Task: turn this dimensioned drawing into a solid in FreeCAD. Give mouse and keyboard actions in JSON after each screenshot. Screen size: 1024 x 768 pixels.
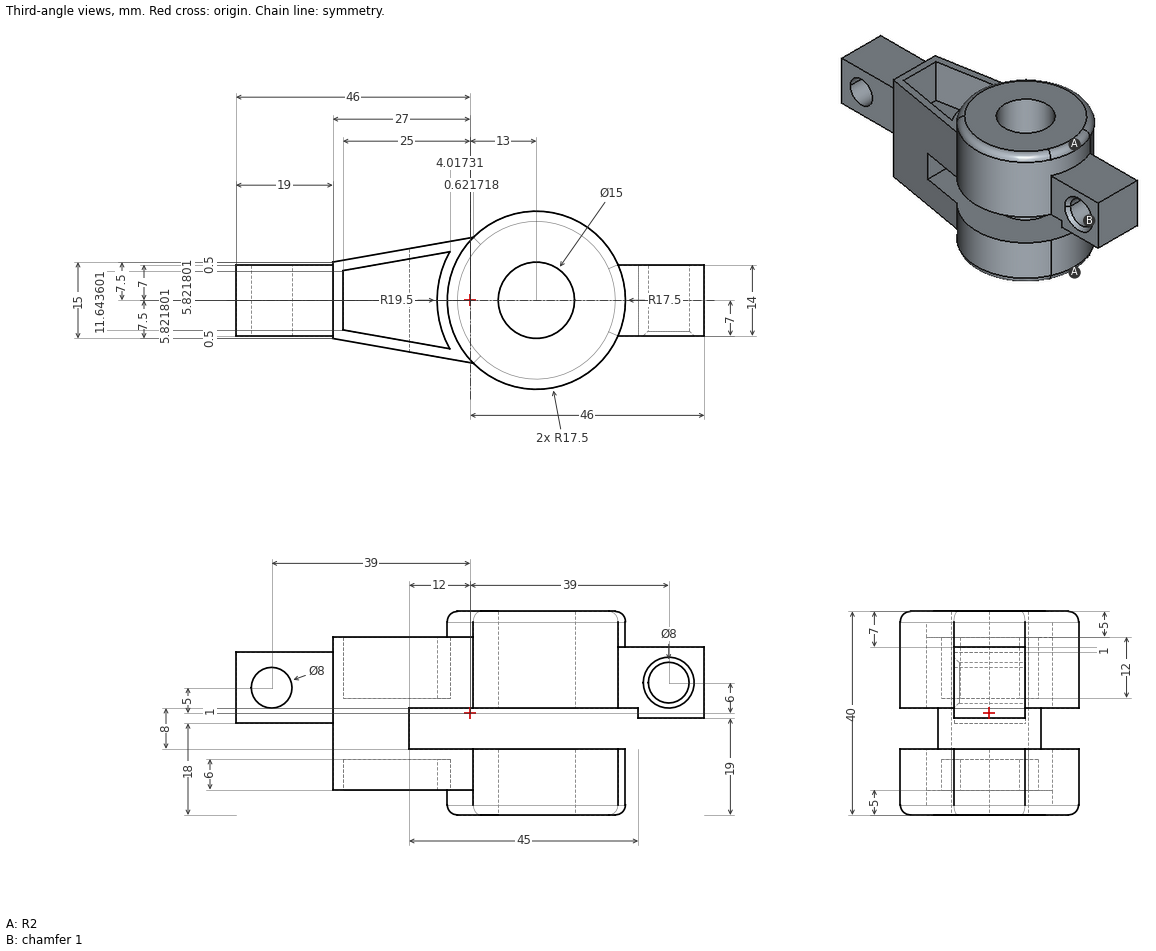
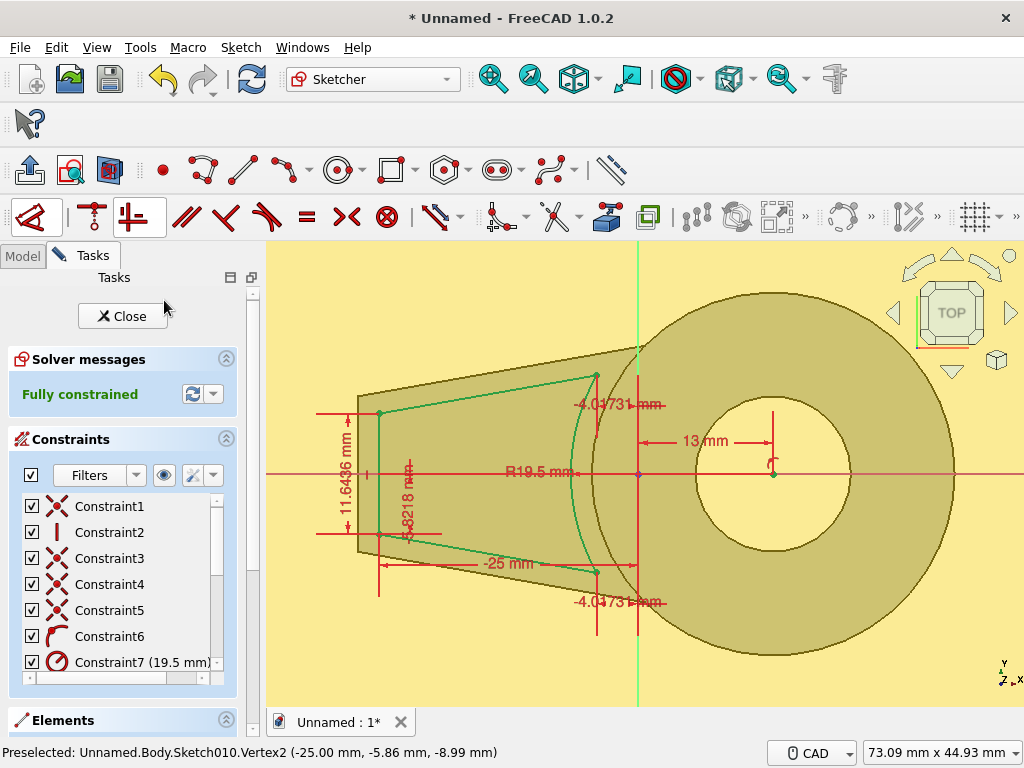
{"action": "left_click", "coordinate": [123, 316]}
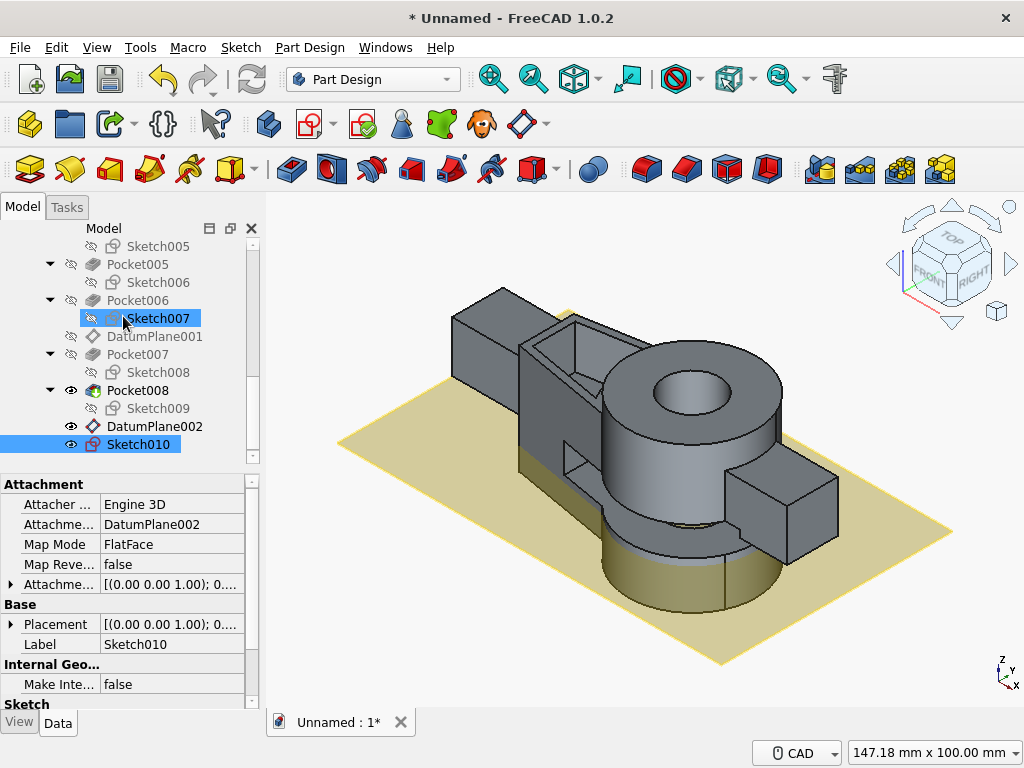
{"action": "left_click", "coordinate": [292, 170]}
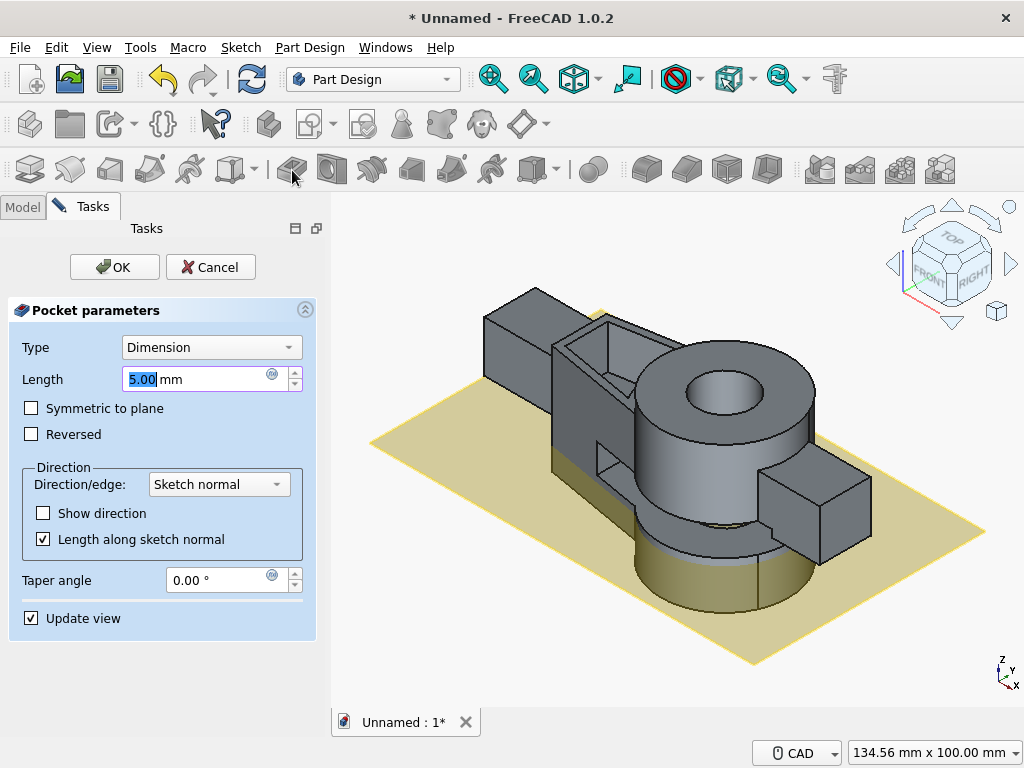
{"action": "type", "text": "6"}
{"action": "key", "text": "Tab"}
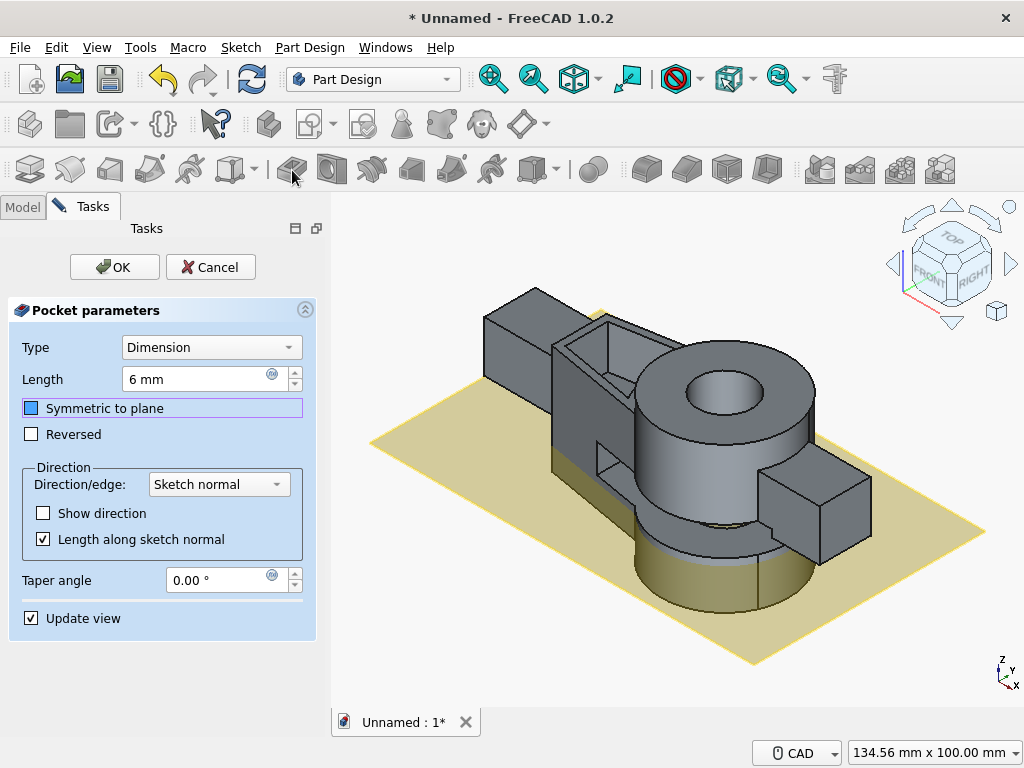
{"action": "left_click", "coordinate": [115, 267]}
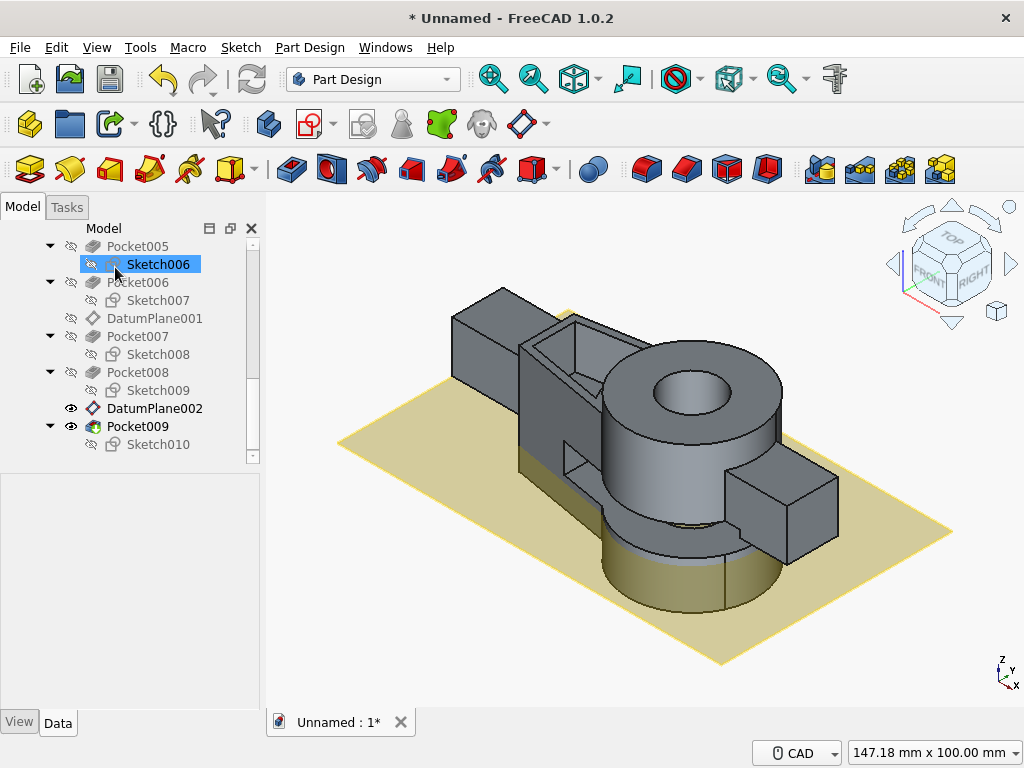
{"action": "left_click", "coordinate": [116, 408]}
{"action": "key", "text": "space"}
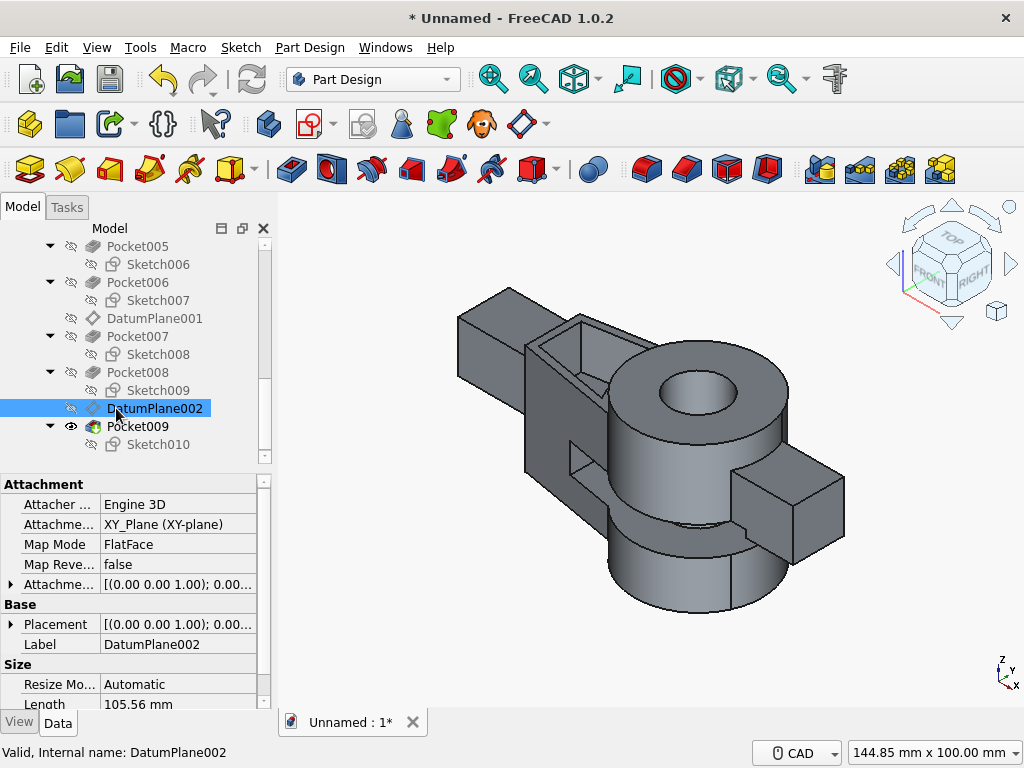
{"action": "left_click", "coordinate": [757, 600]}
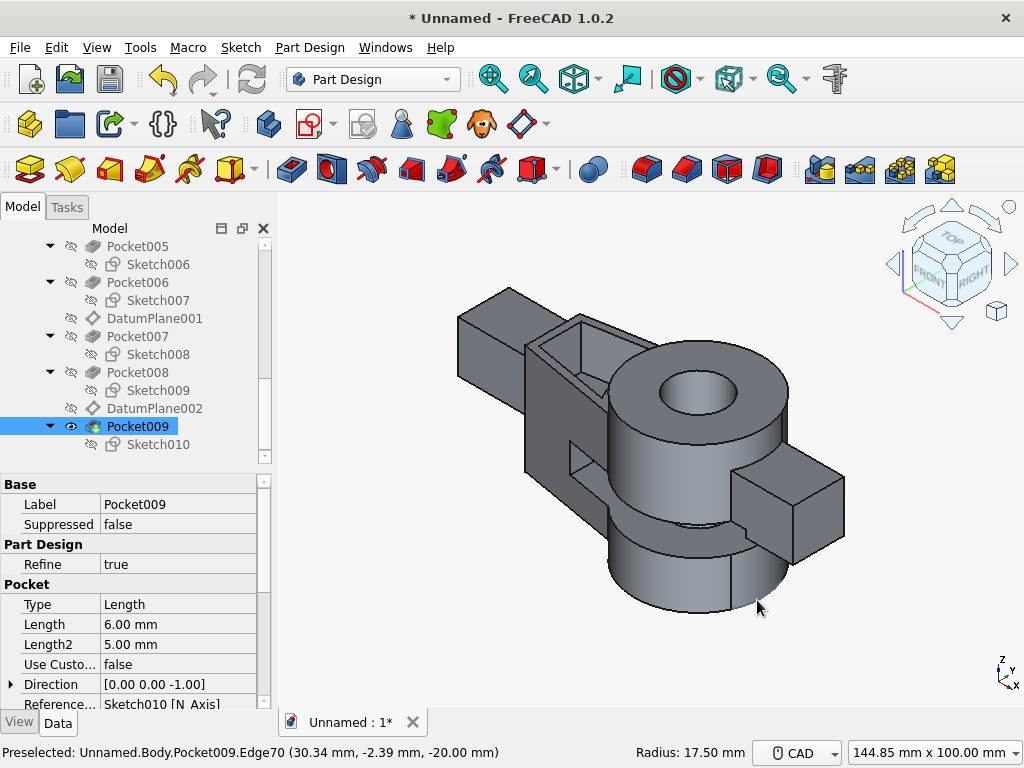
{"action": "left_click", "coordinate": [762, 429], "text": "ctrl"}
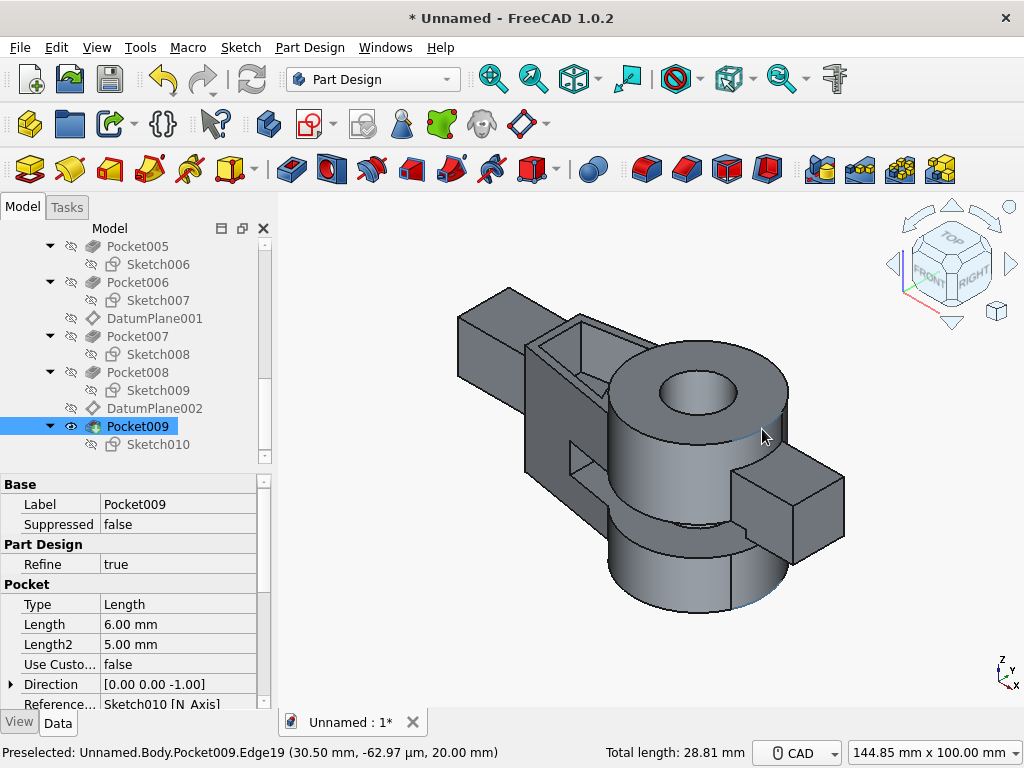
{"action": "left_click", "coordinate": [648, 170]}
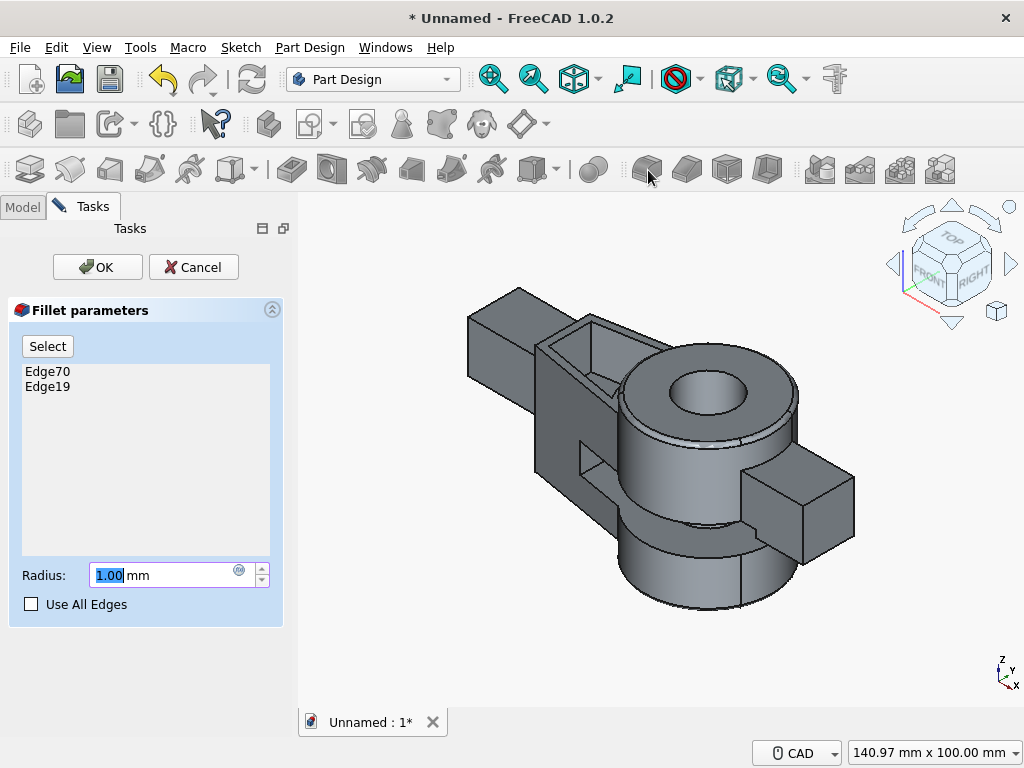
{"action": "type", "text": "2"}
{"action": "key", "text": "Tab"}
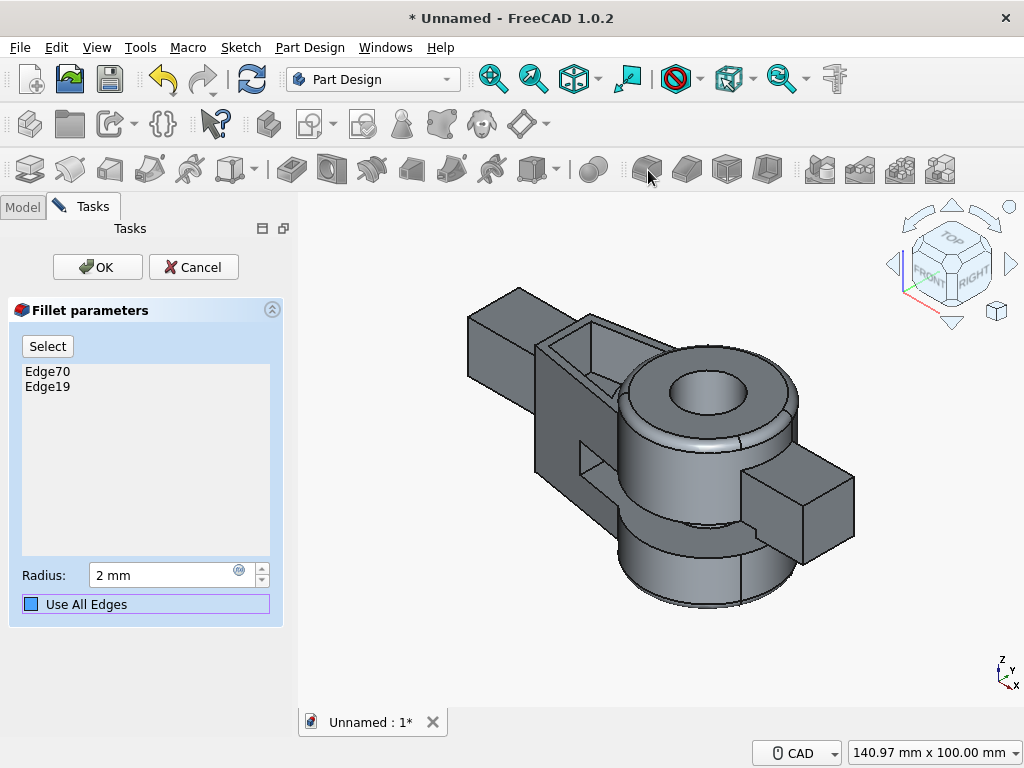
{"action": "left_click", "coordinate": [98, 267]}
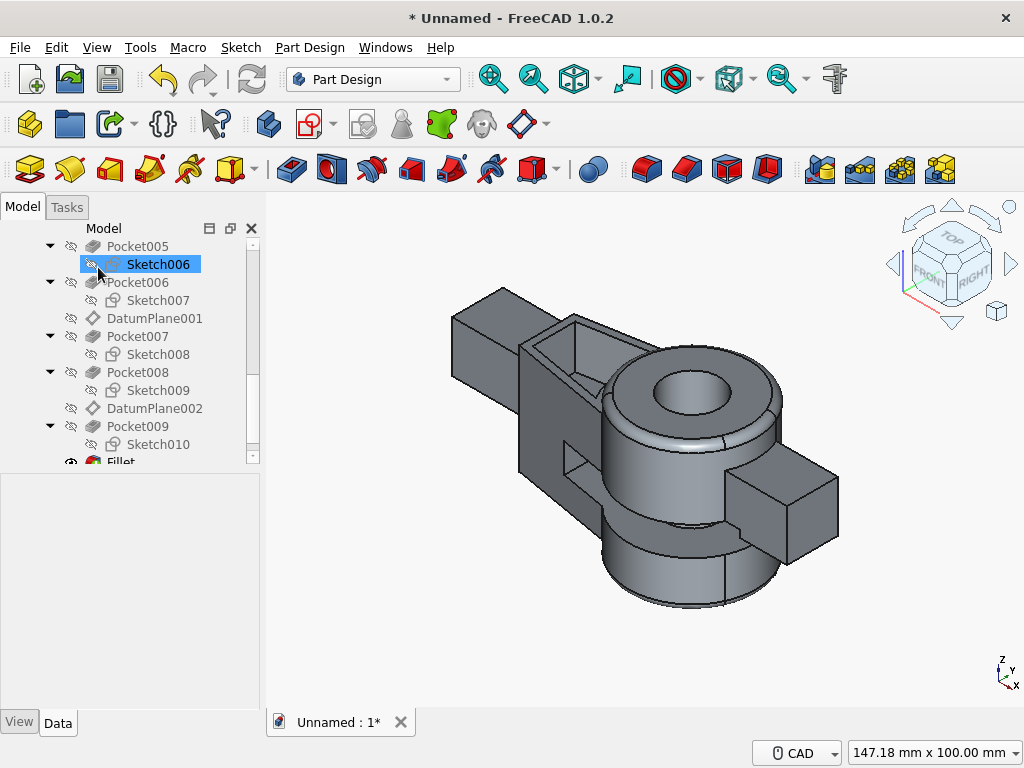
{"action": "key", "text": "4"}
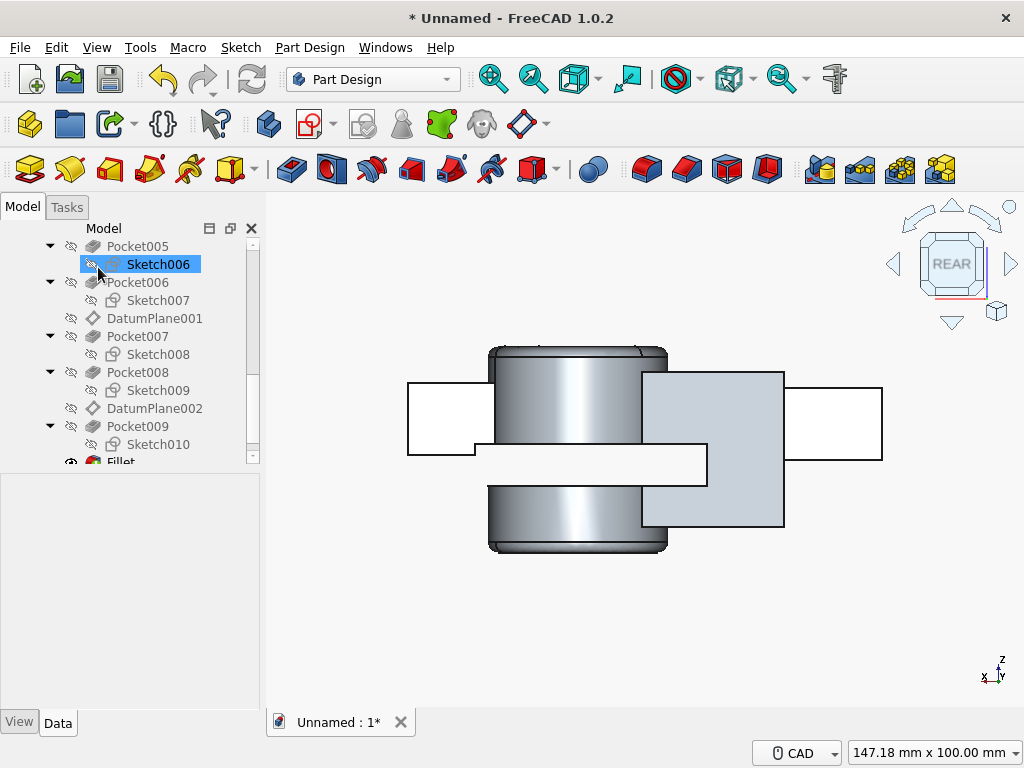
{"action": "left_click", "coordinate": [833, 423]}